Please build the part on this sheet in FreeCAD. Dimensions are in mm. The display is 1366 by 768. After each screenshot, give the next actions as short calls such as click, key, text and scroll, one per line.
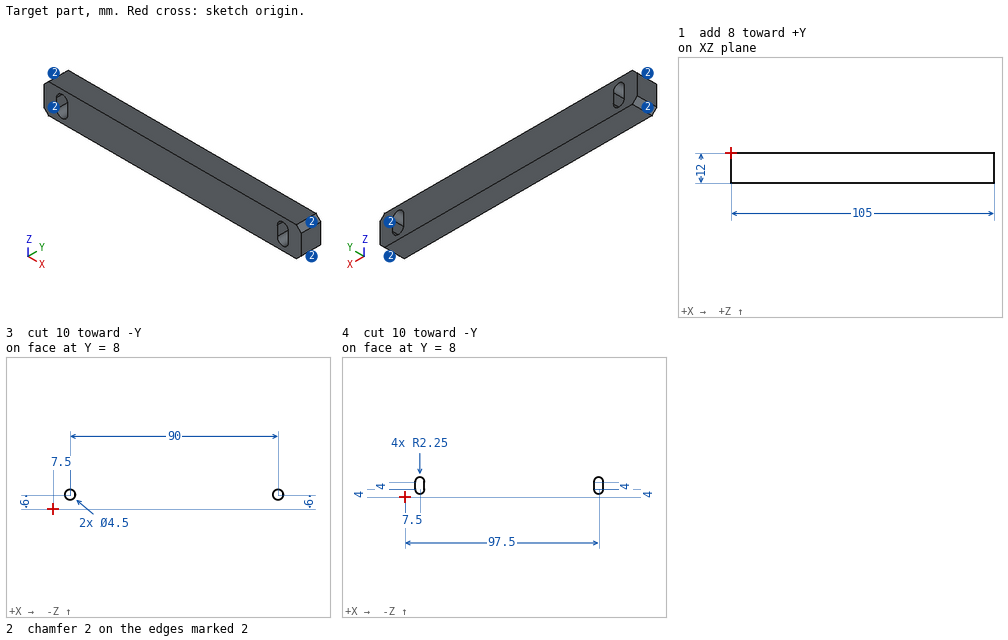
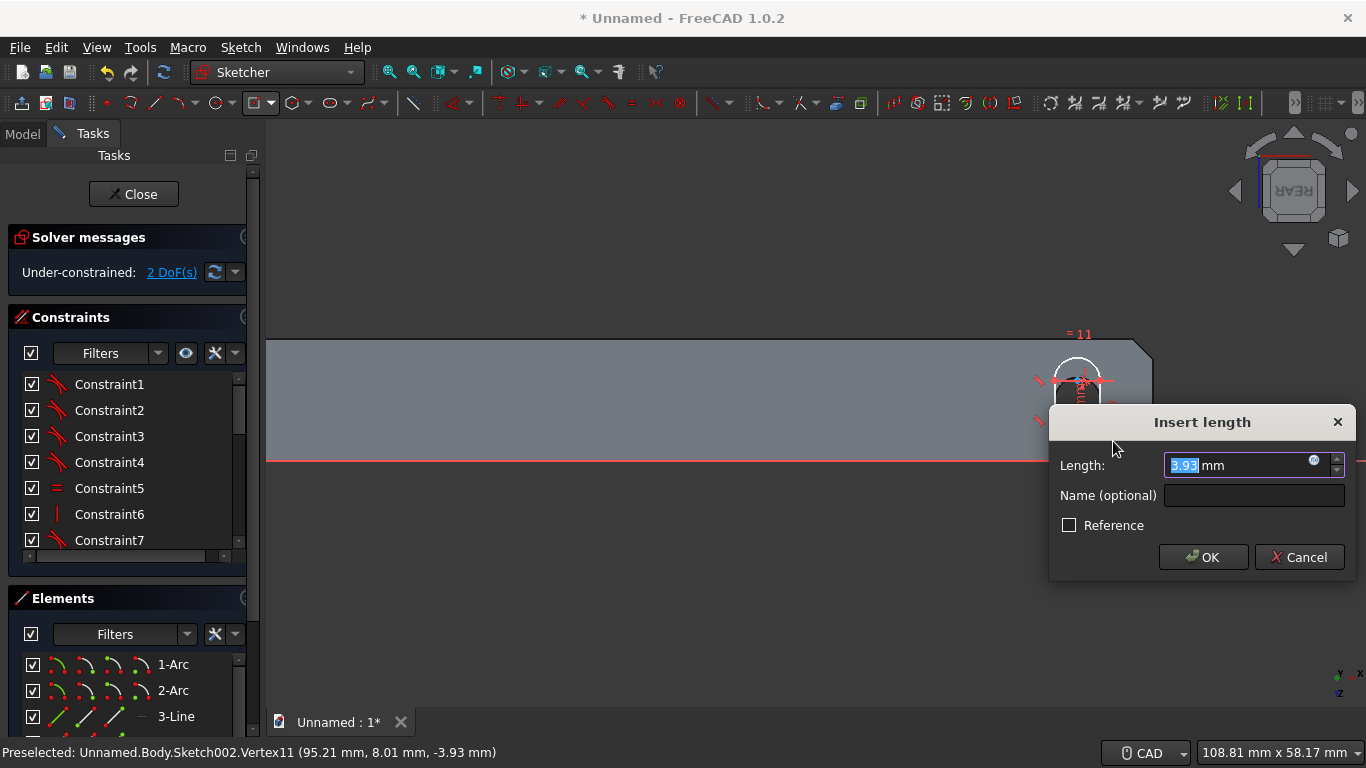
text(4)
key(Return)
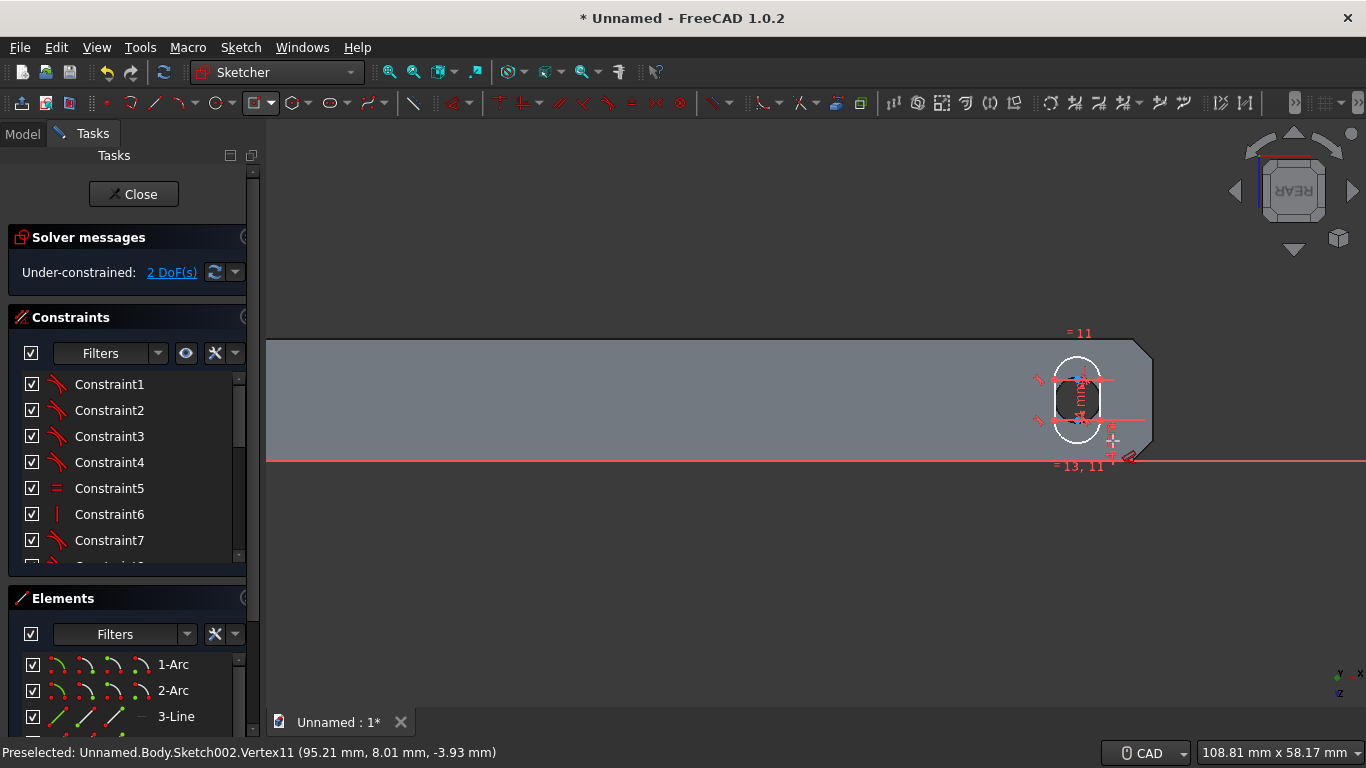
scroll(1055, 421, down, 2)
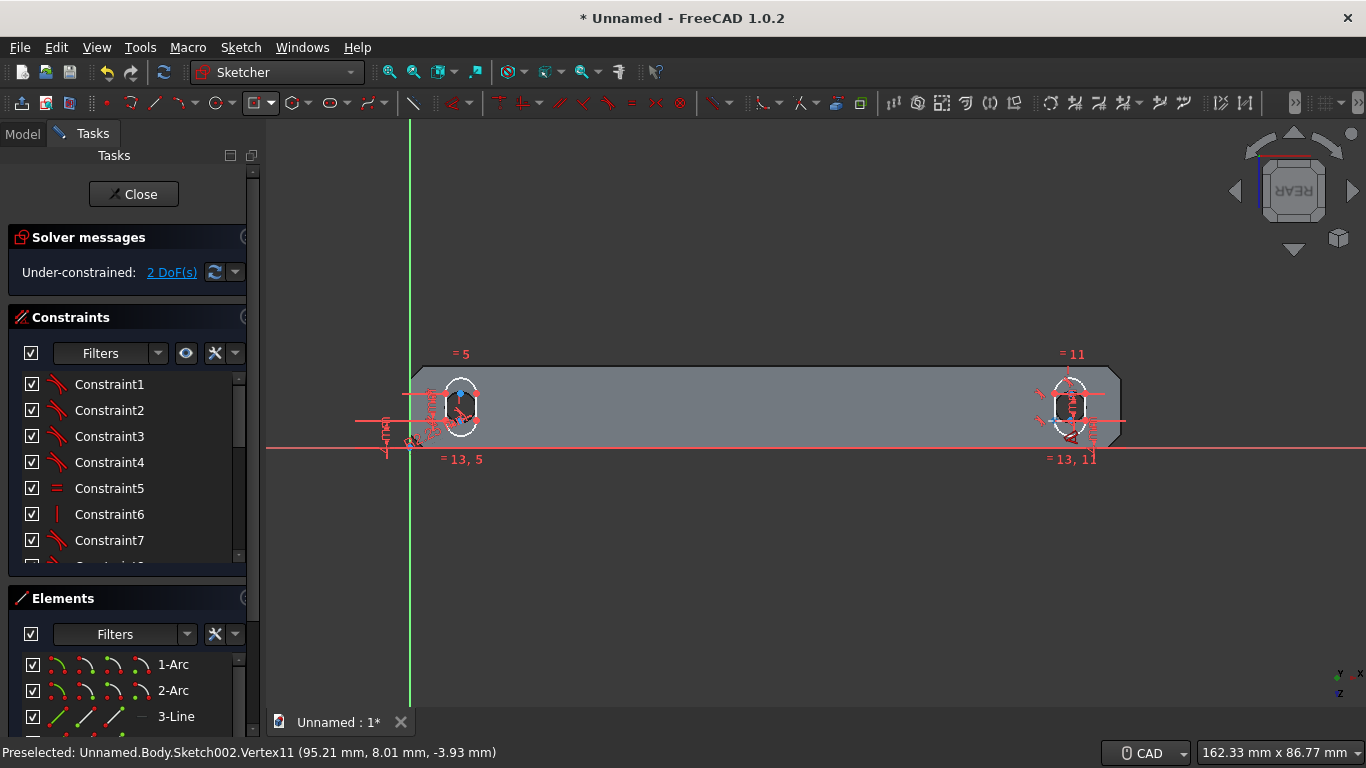
click(461, 421)
click(435, 482)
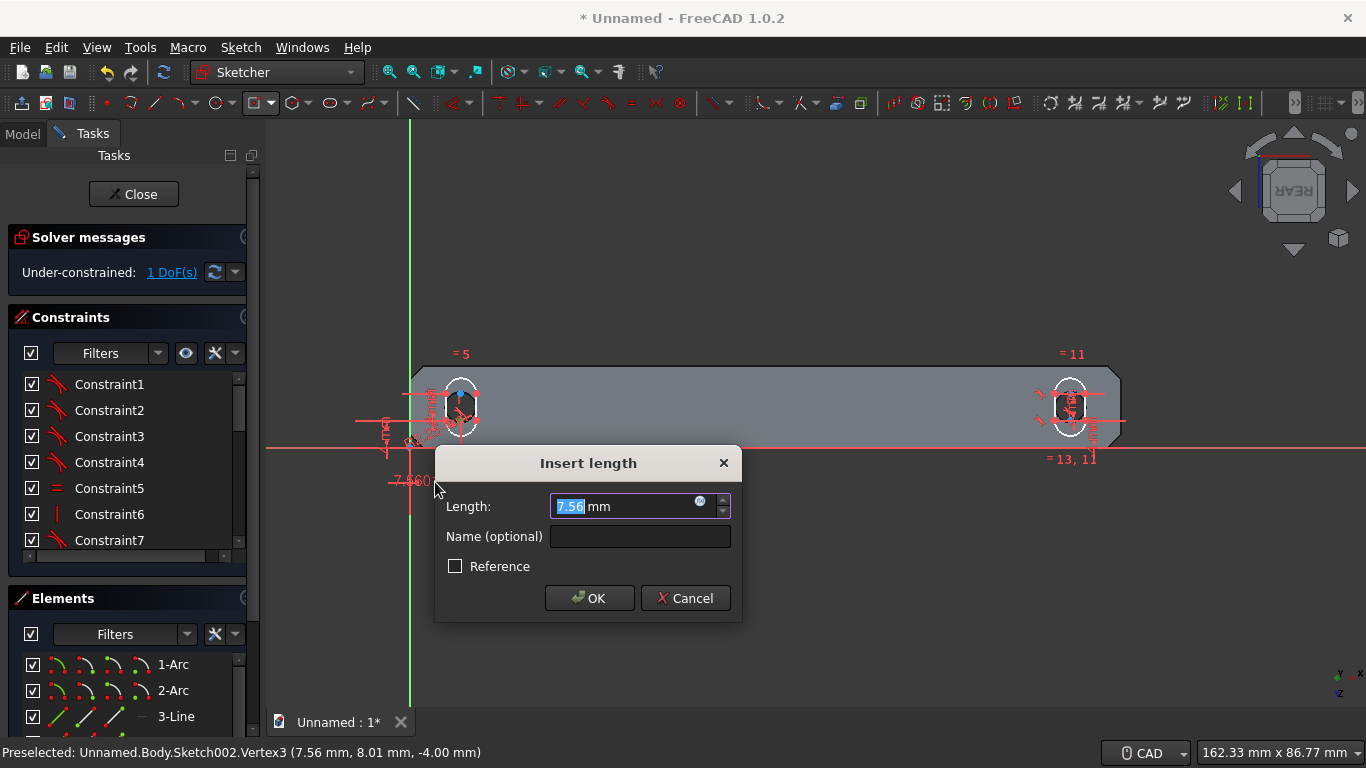
text(7.5)
key(Return)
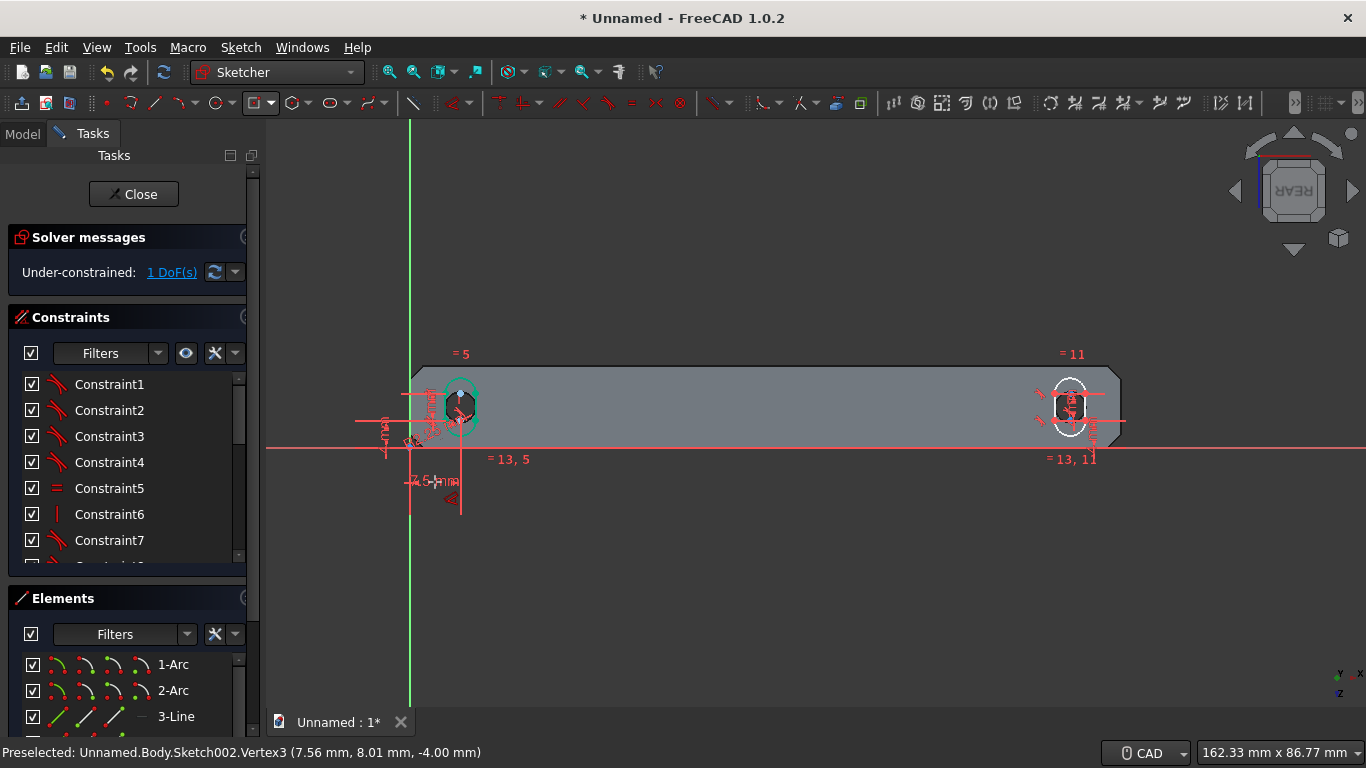
click(1070, 421)
click(740, 482)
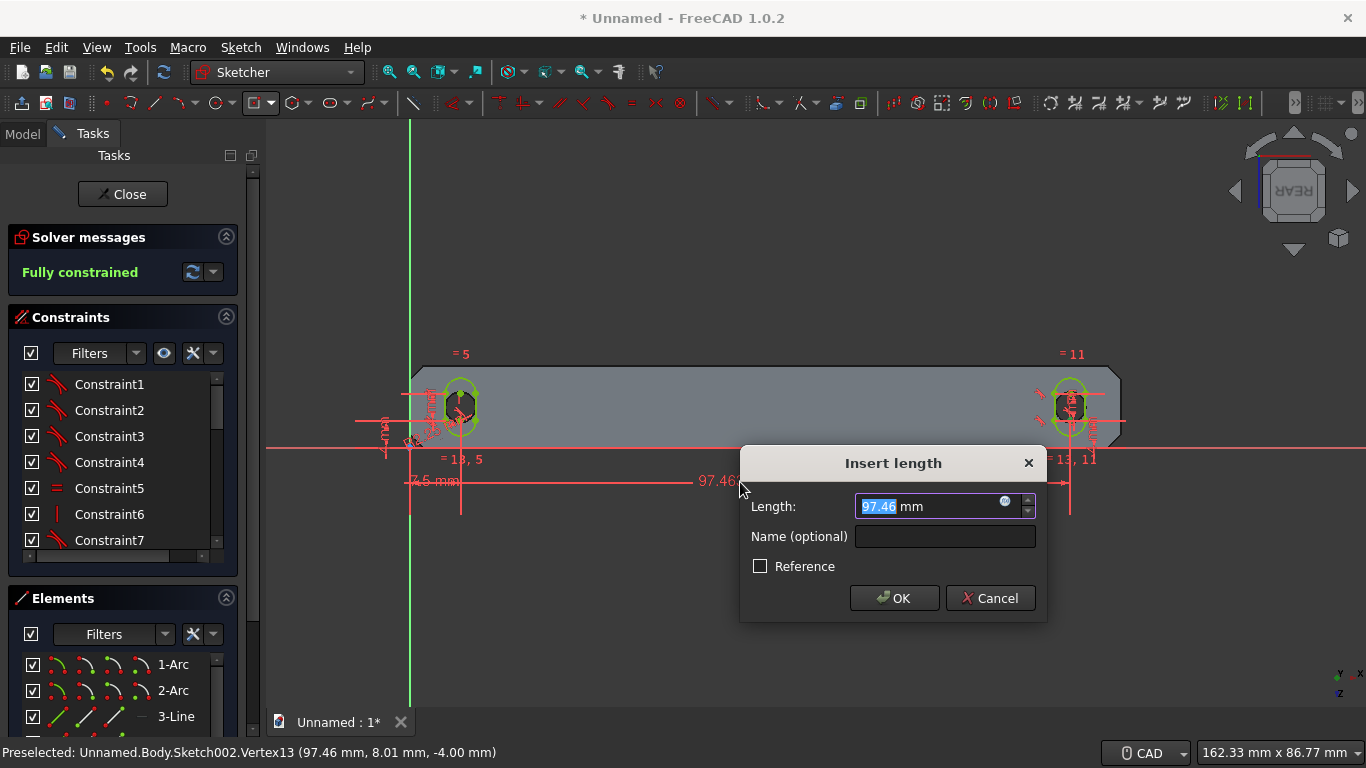
text(97.5)
key(Return)
key(Escape)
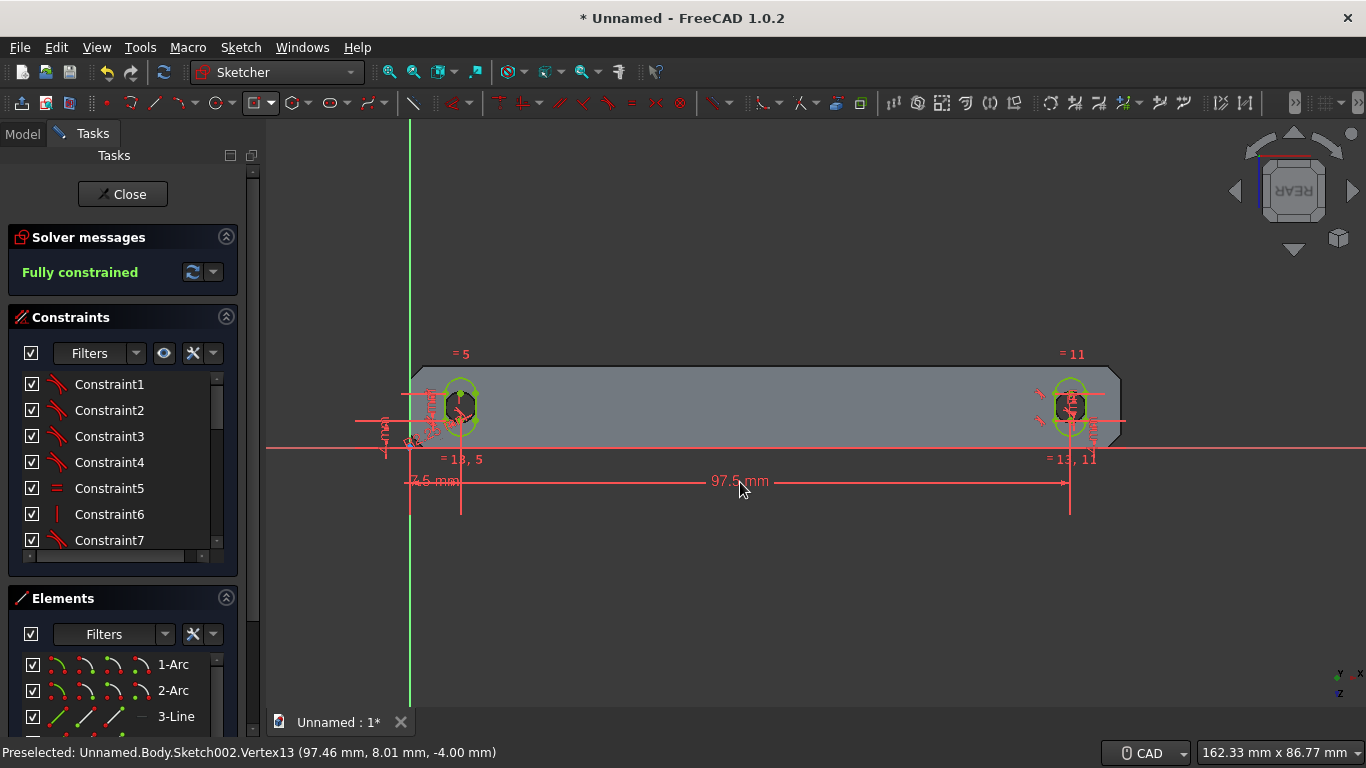
click(123, 194)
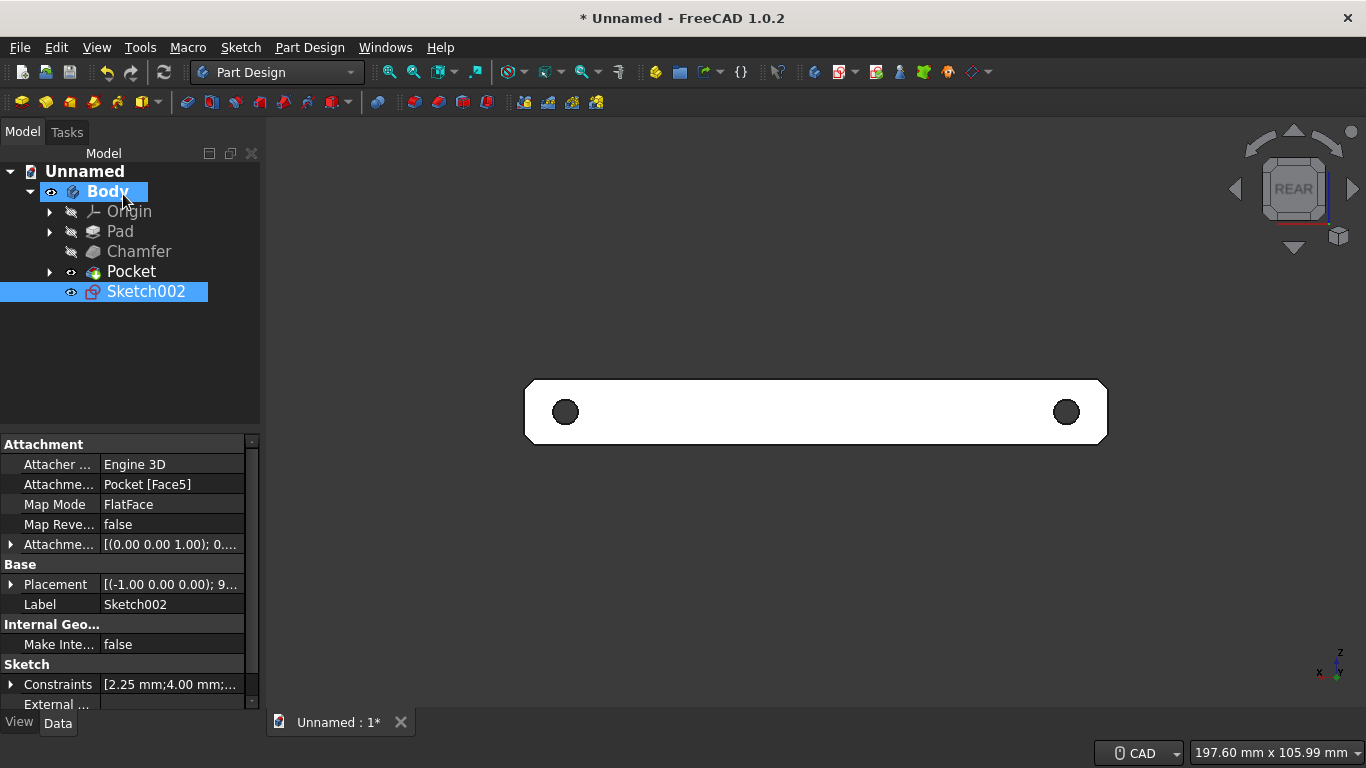
click(188, 102)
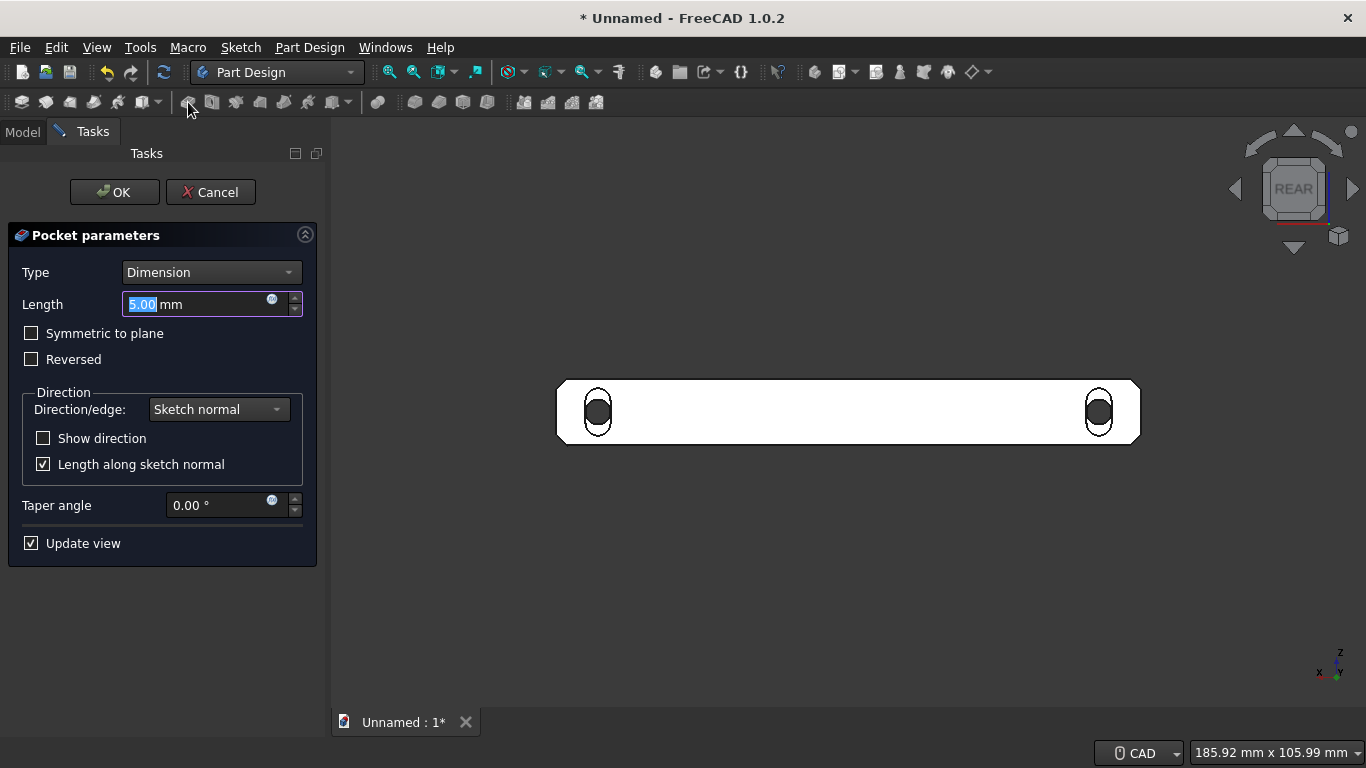
text(10)
key(Tab)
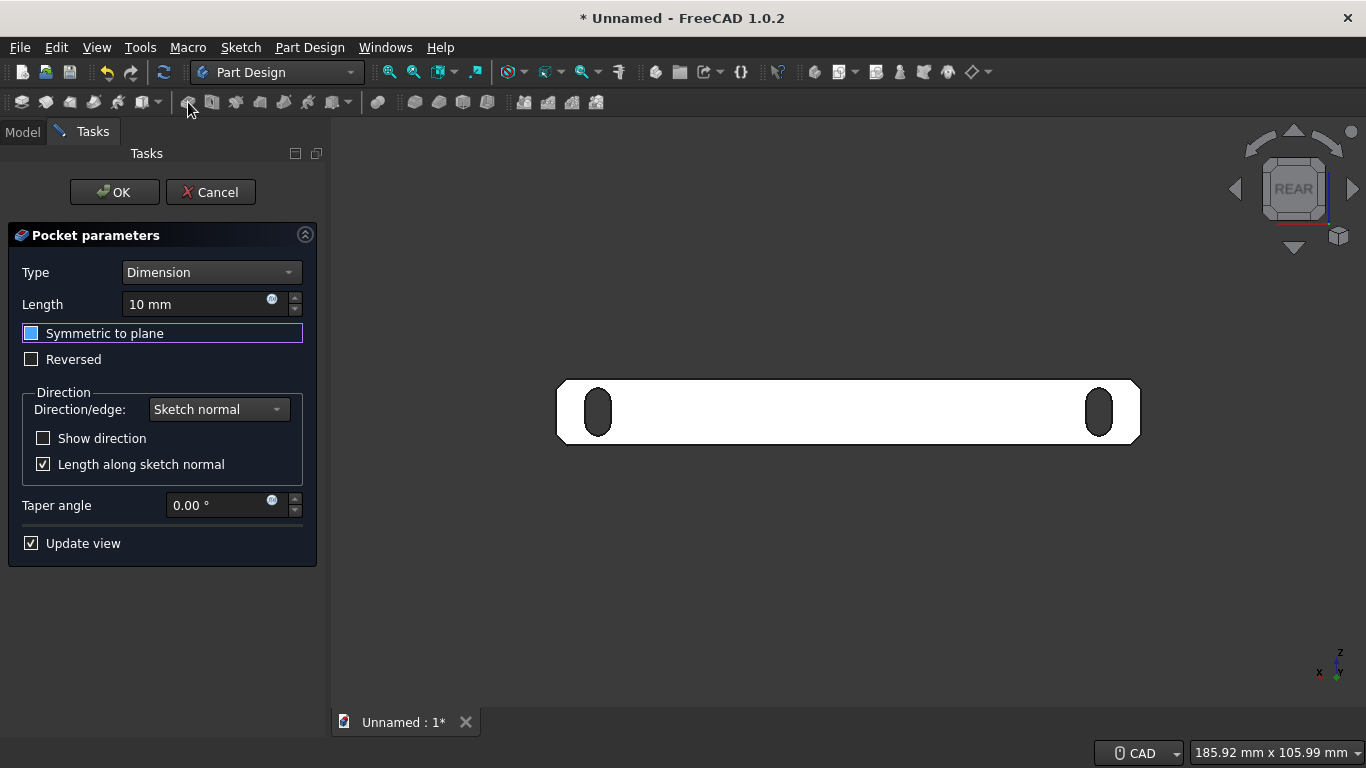
click(115, 192)